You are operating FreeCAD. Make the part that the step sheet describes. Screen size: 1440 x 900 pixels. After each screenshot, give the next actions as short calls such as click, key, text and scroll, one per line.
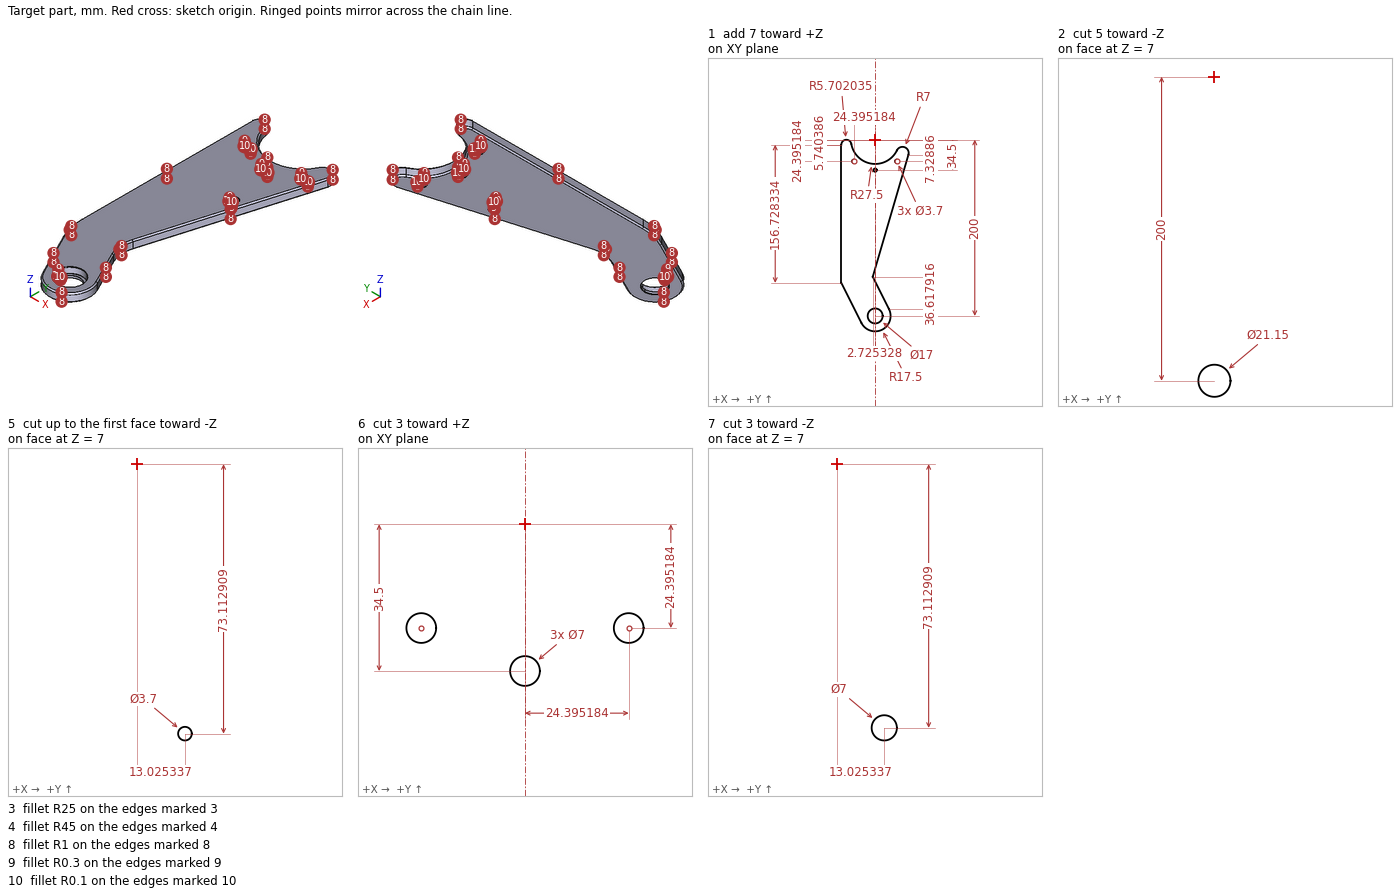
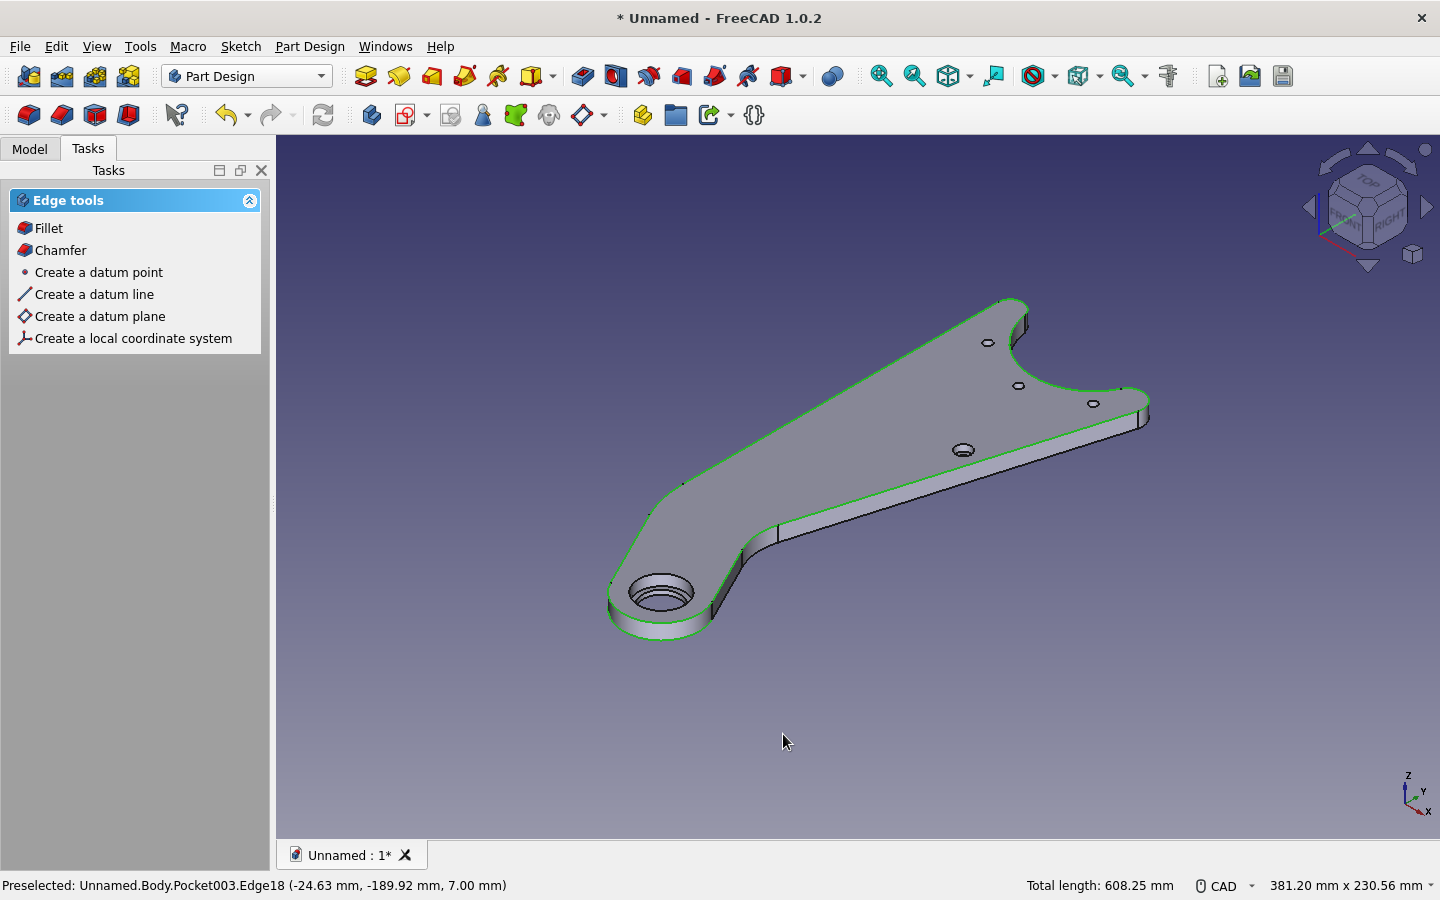
key(1)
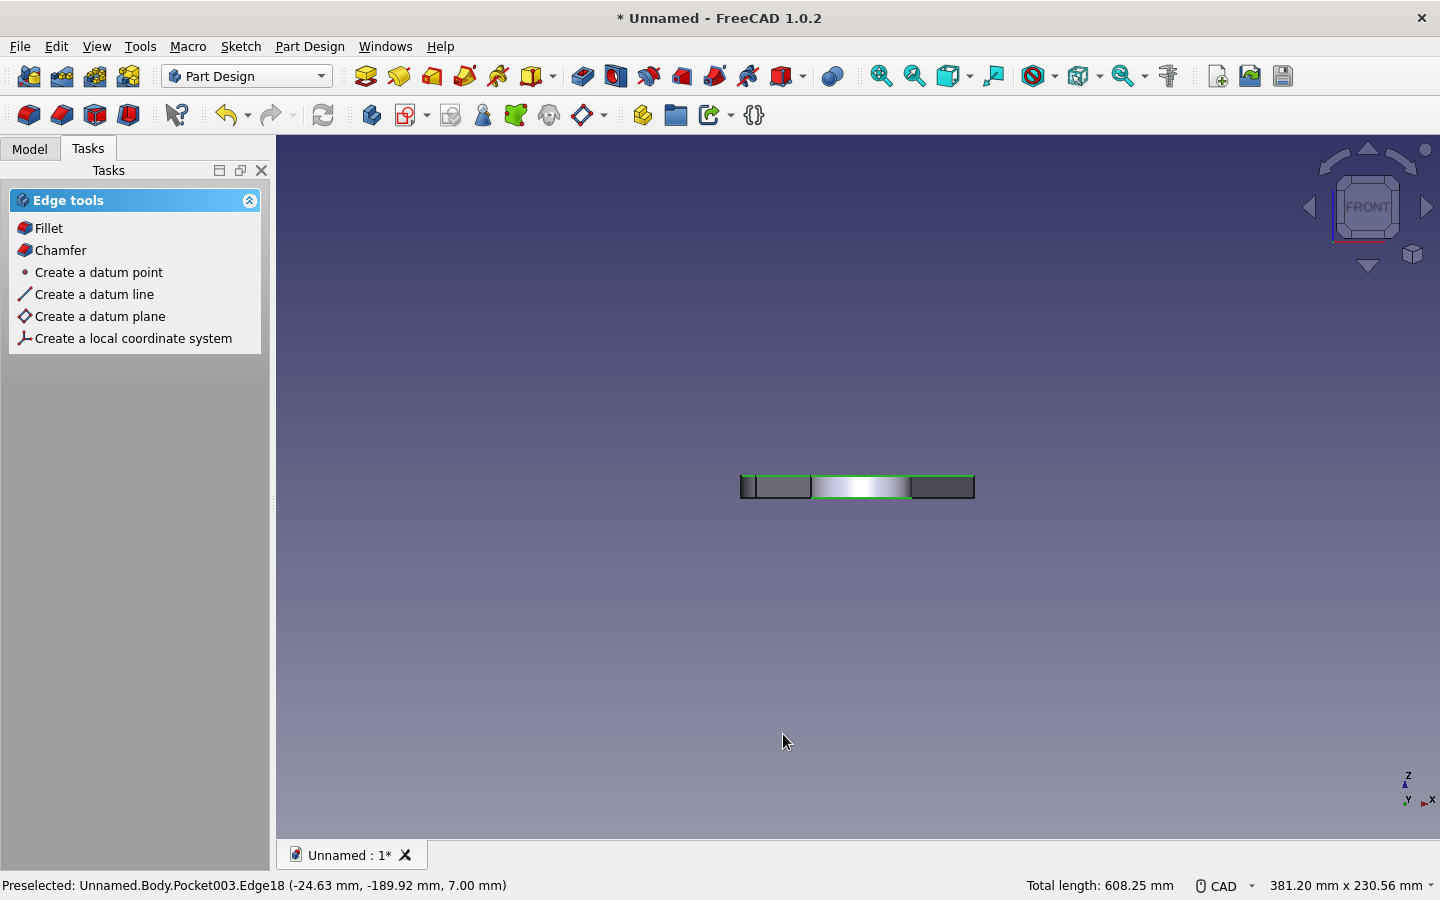
click(882, 76)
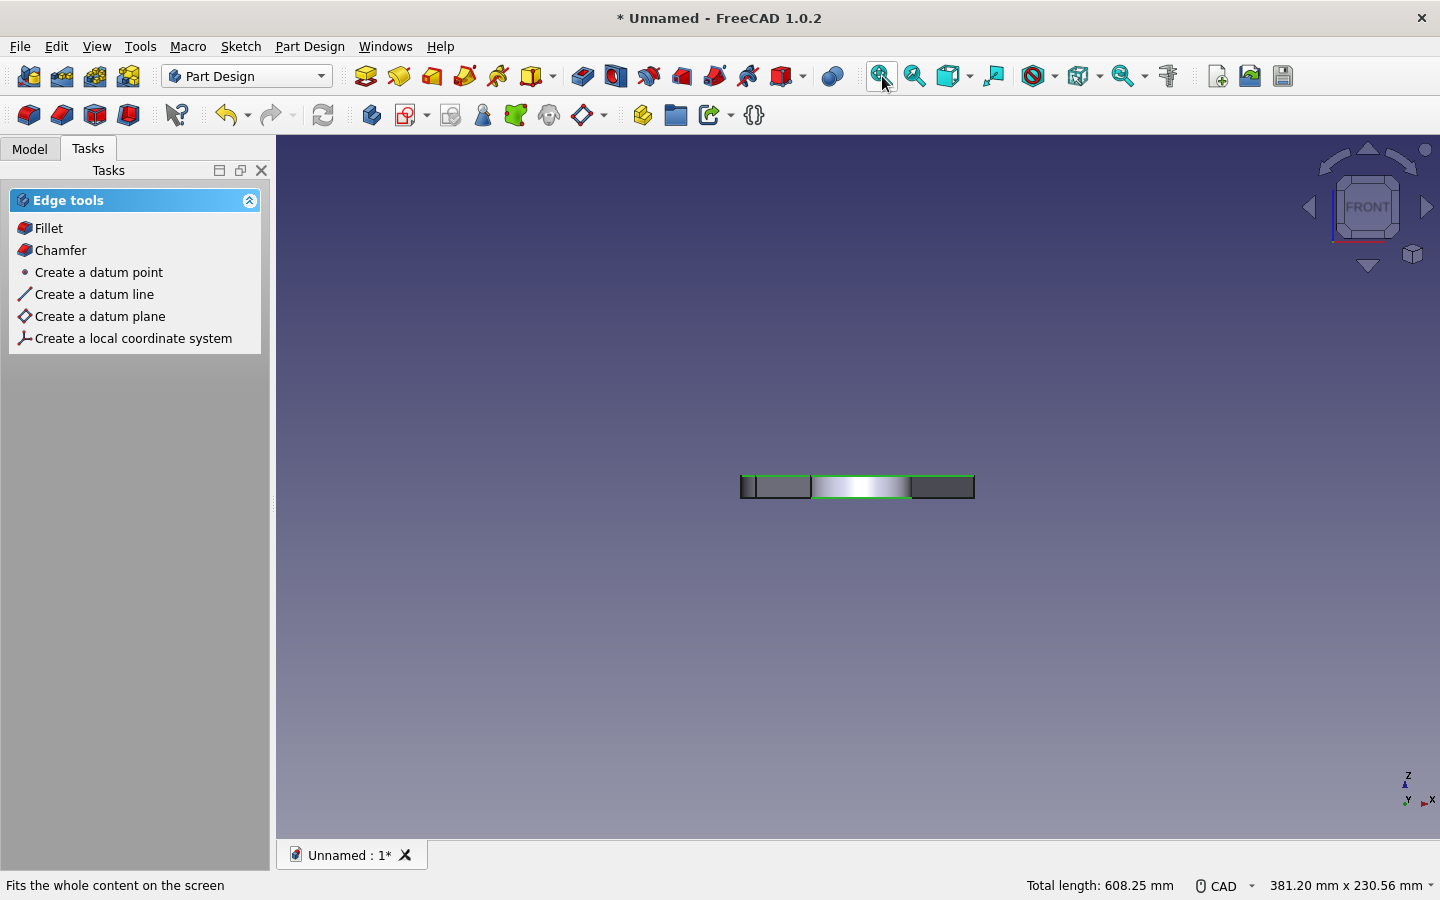
click(916, 497, ctrl)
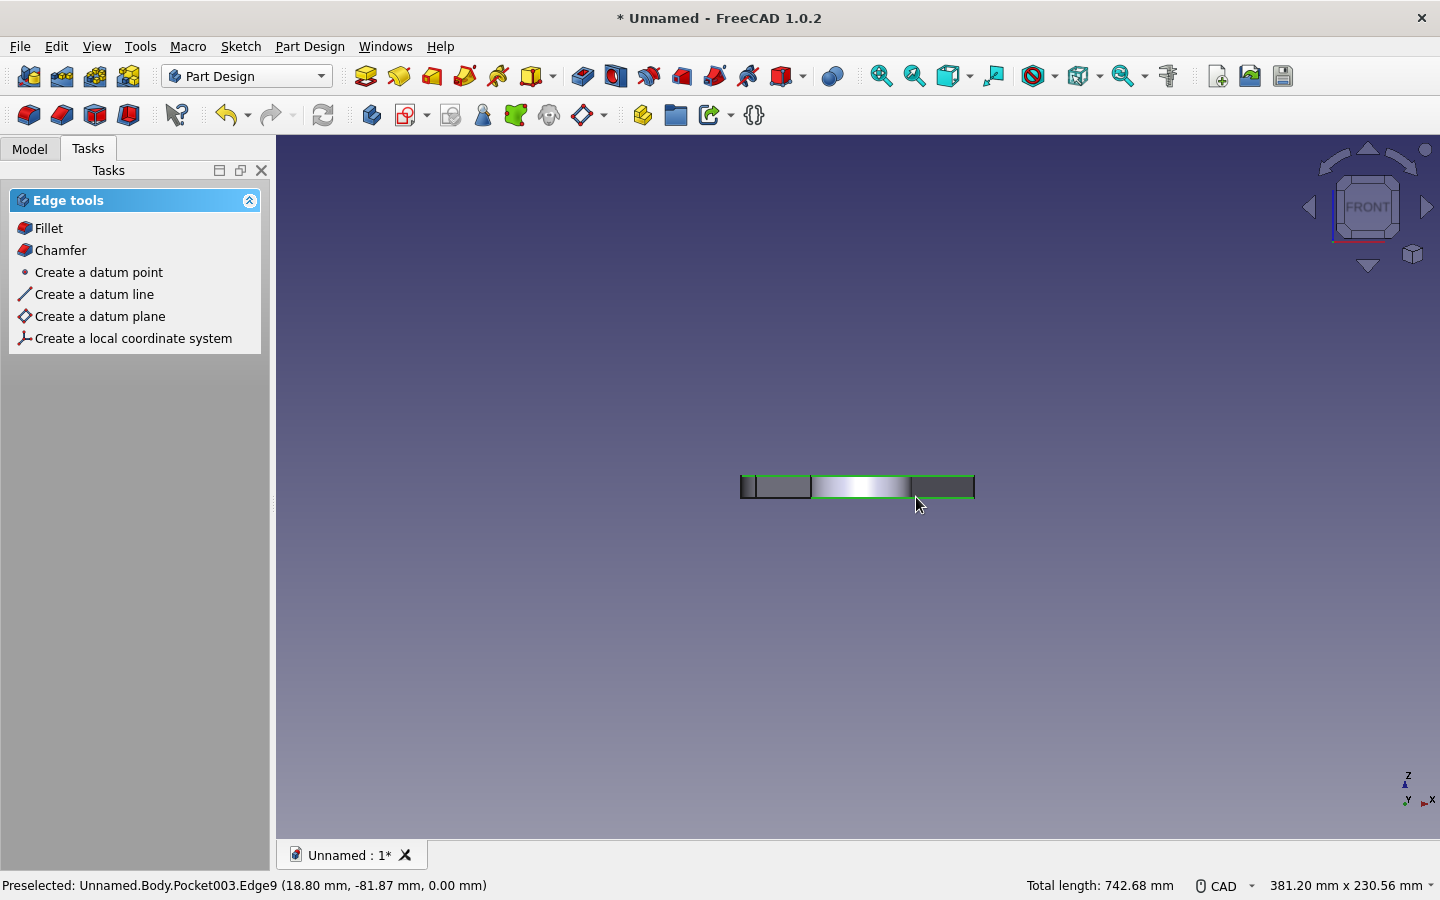
click(783, 497, ctrl)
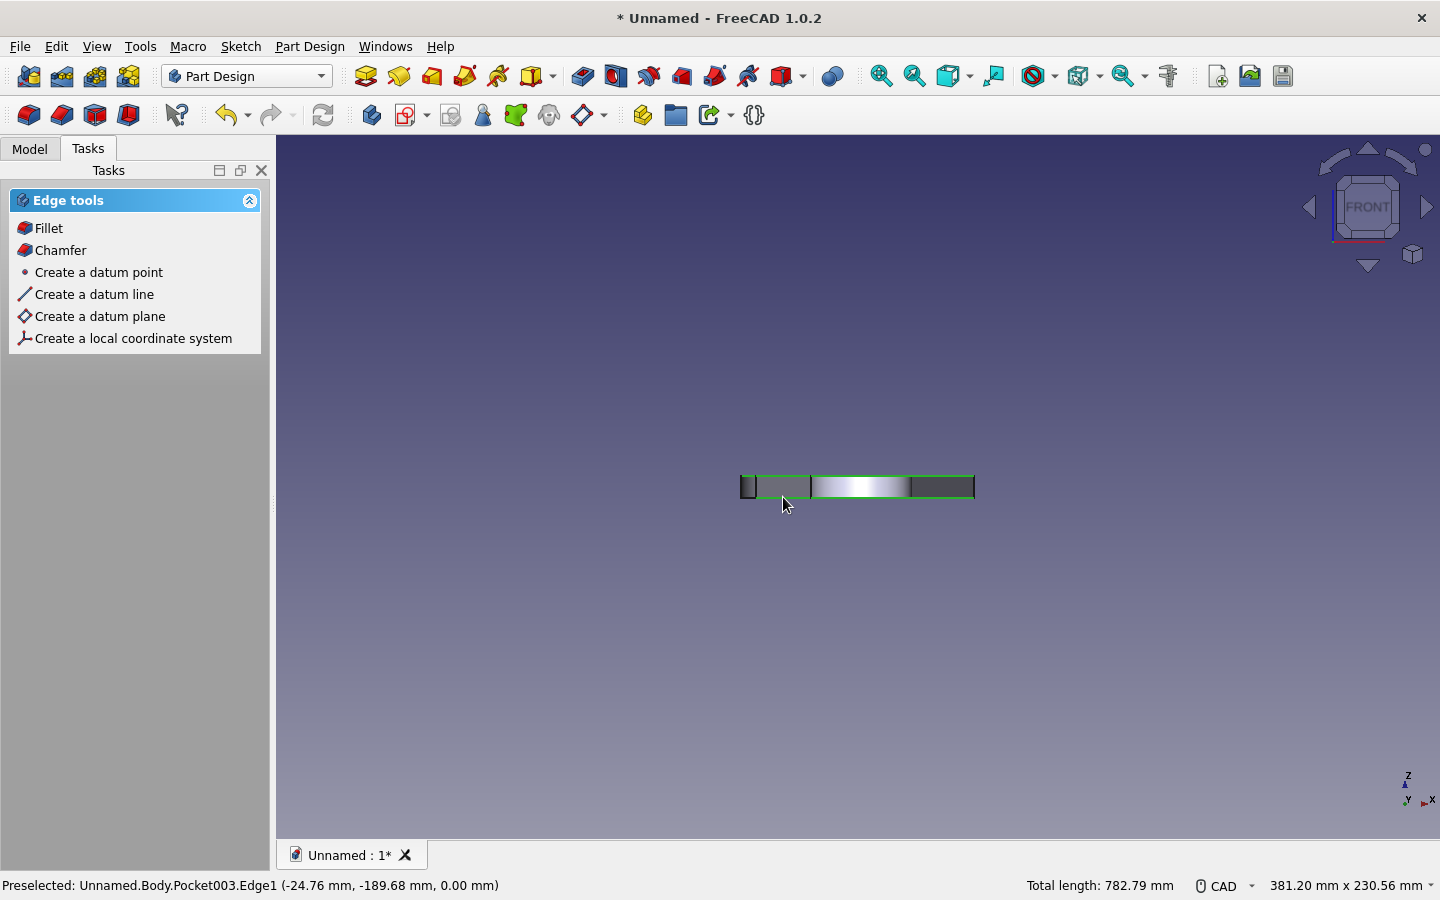
click(745, 497, ctrl)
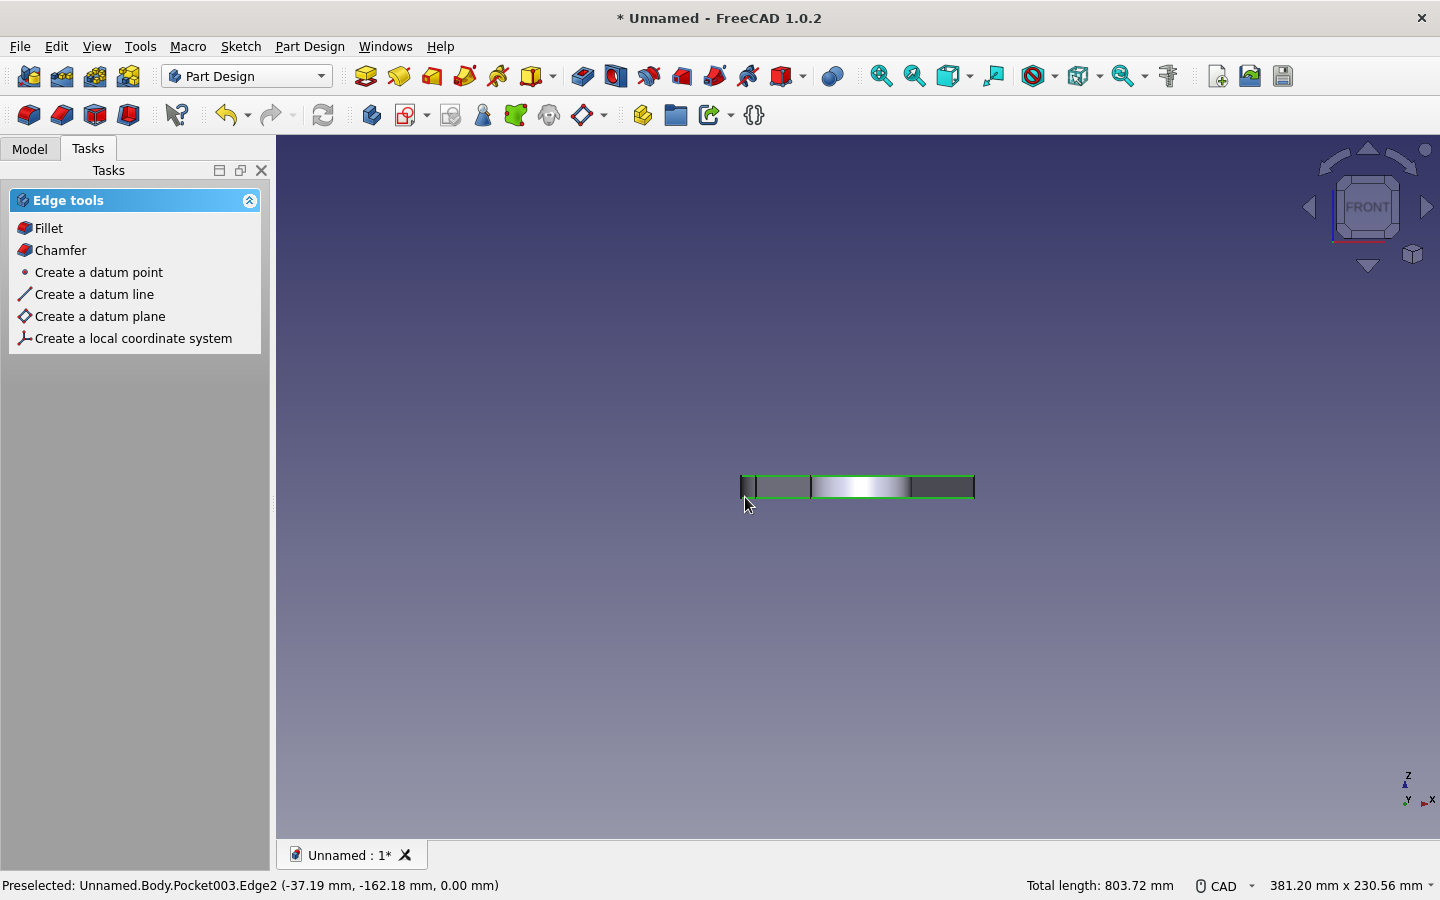
key(3)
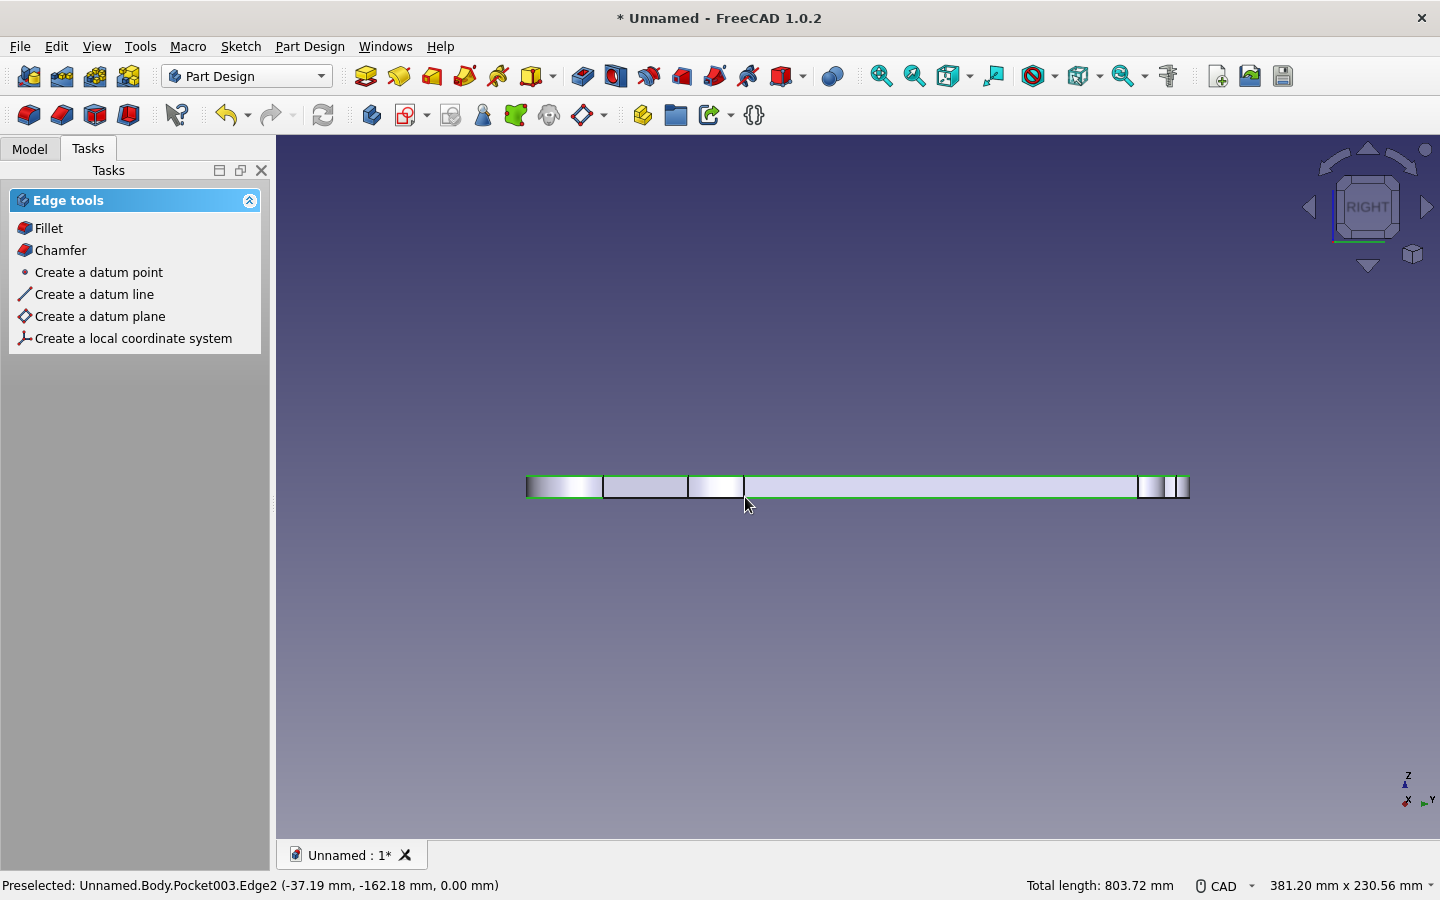
click(1190, 497, ctrl)